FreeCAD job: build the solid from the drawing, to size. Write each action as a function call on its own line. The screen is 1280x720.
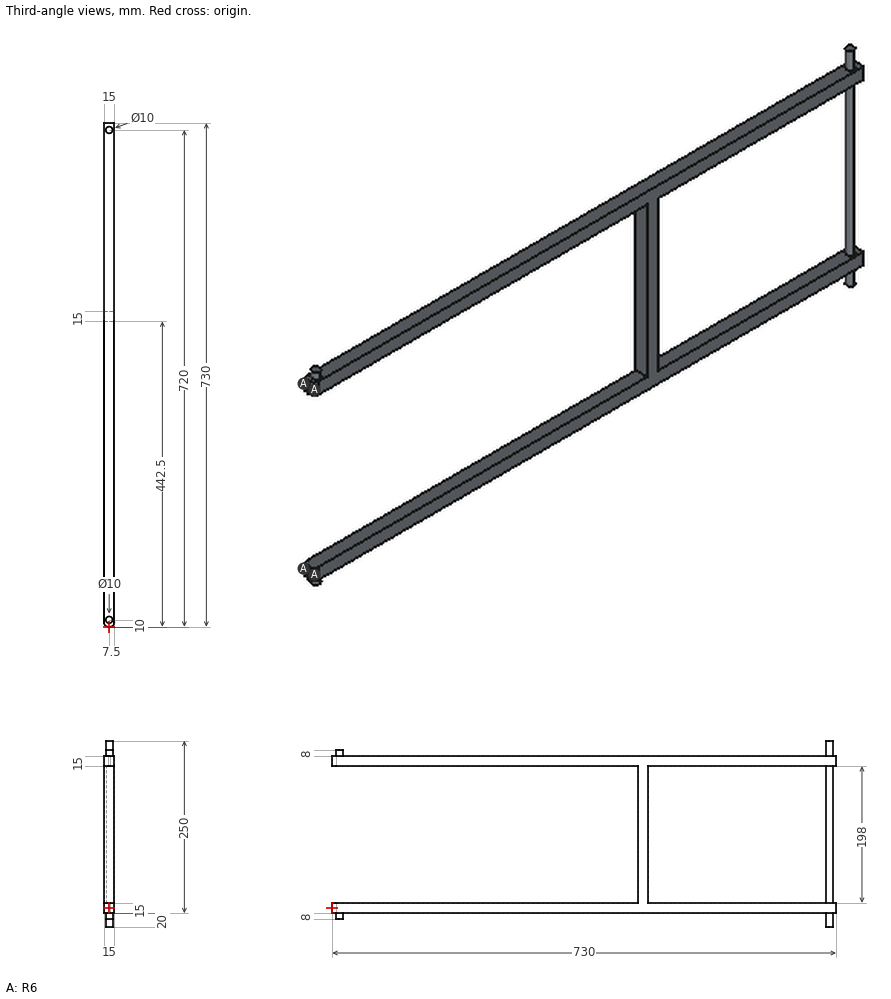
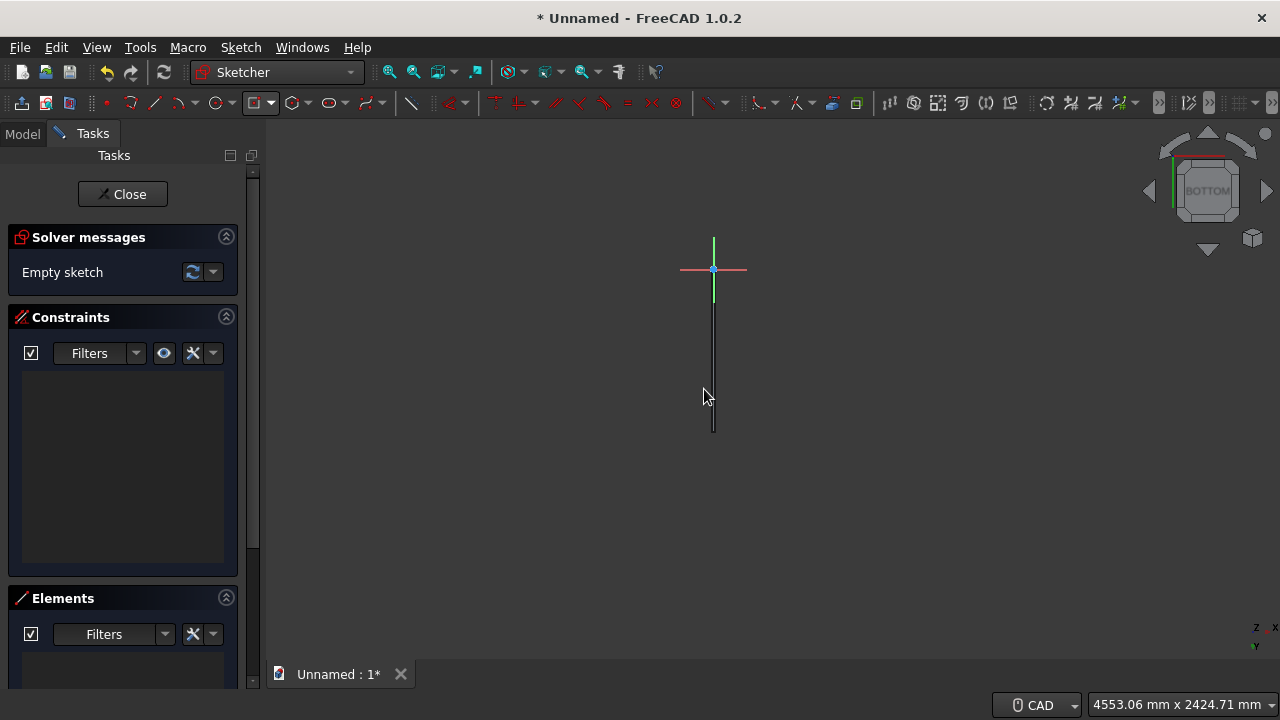
scroll(714, 265, up, 15)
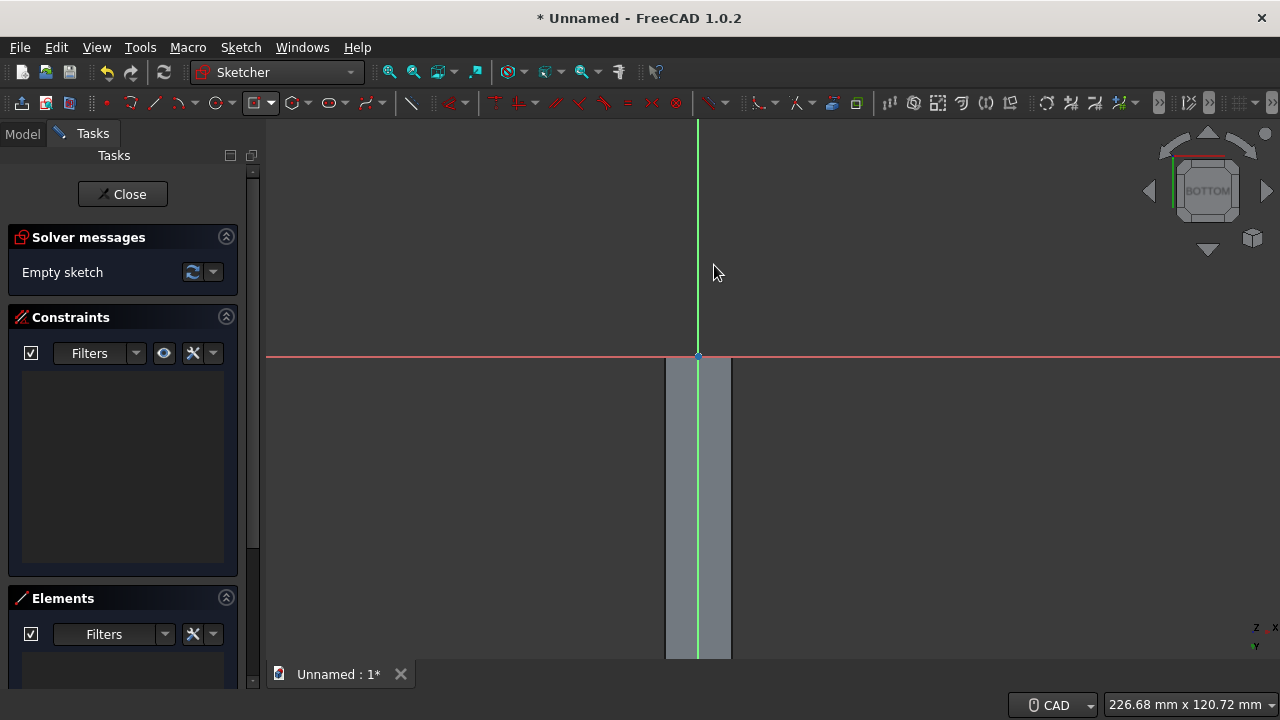
scroll(696, 390, up, 8)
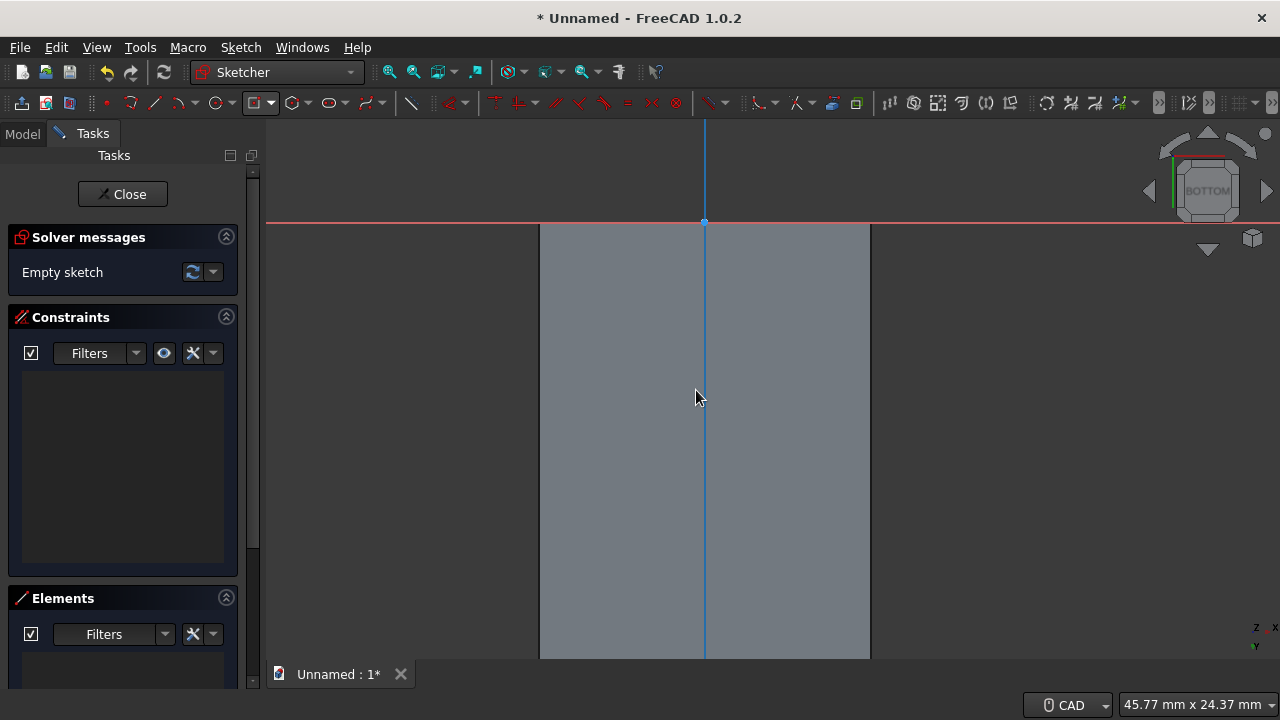
click(216, 104)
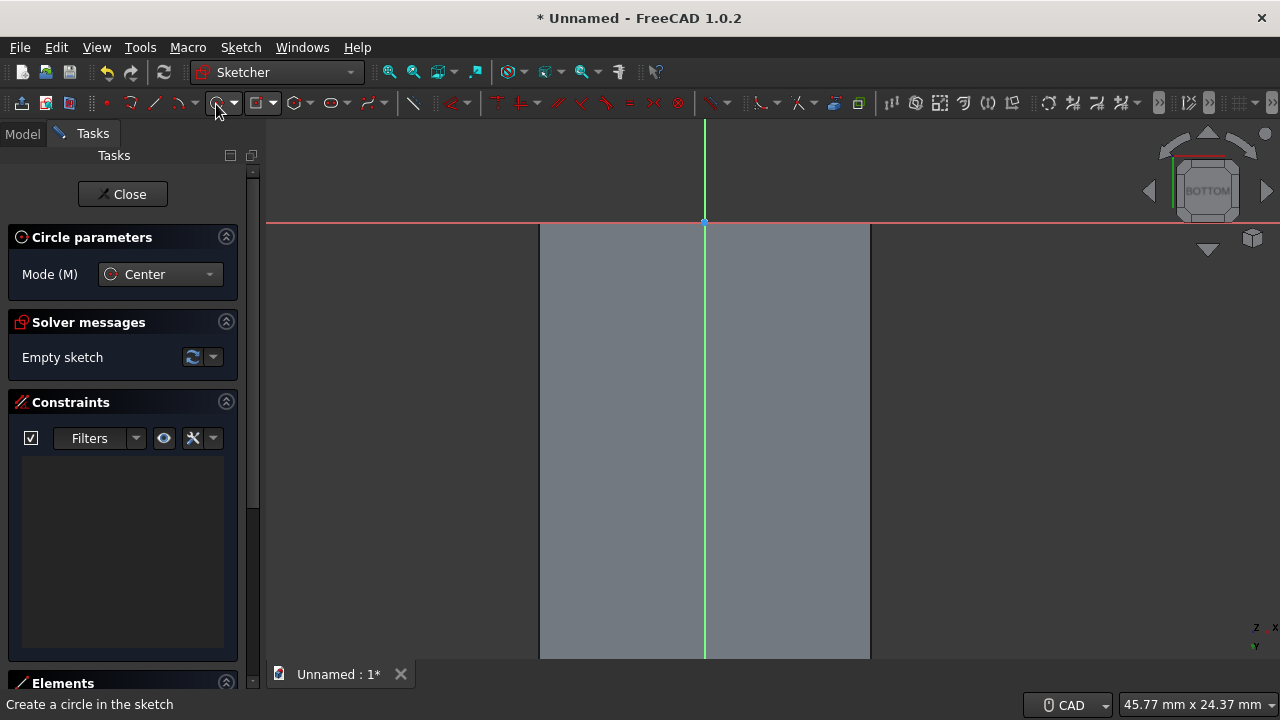
click(705, 444)
move(783, 366)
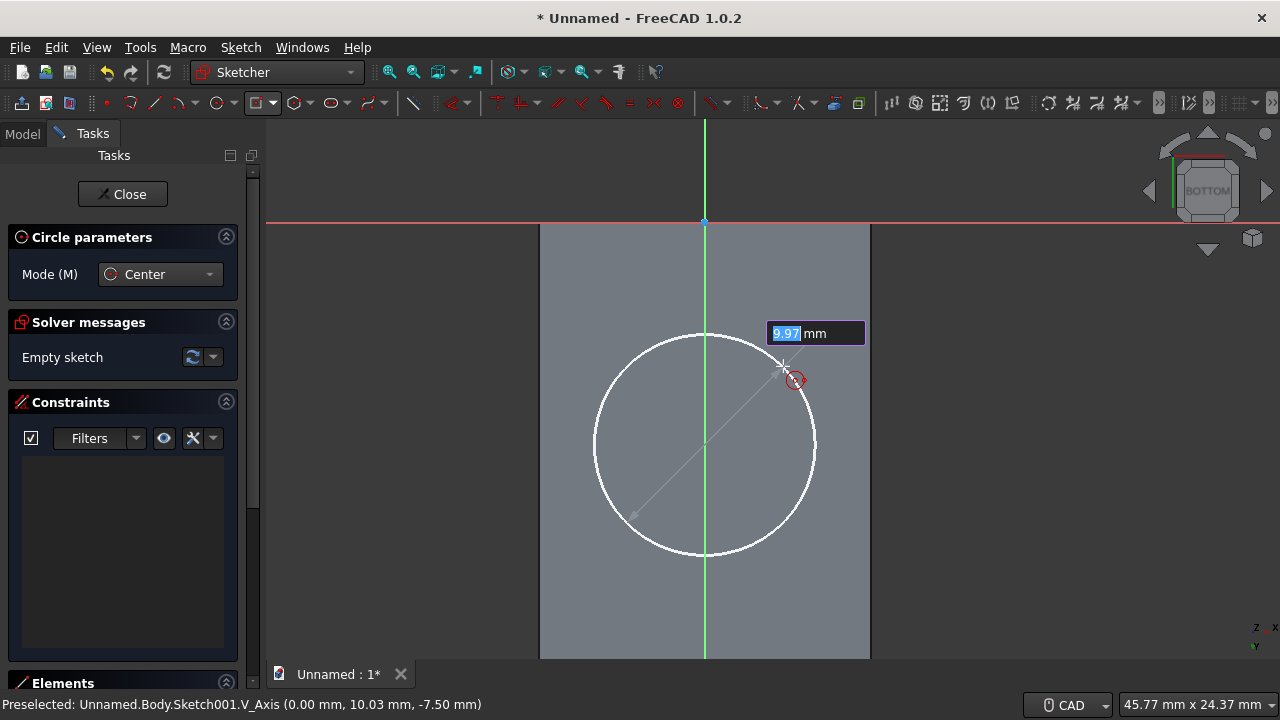
text(10)
key(Return)
key(Escape)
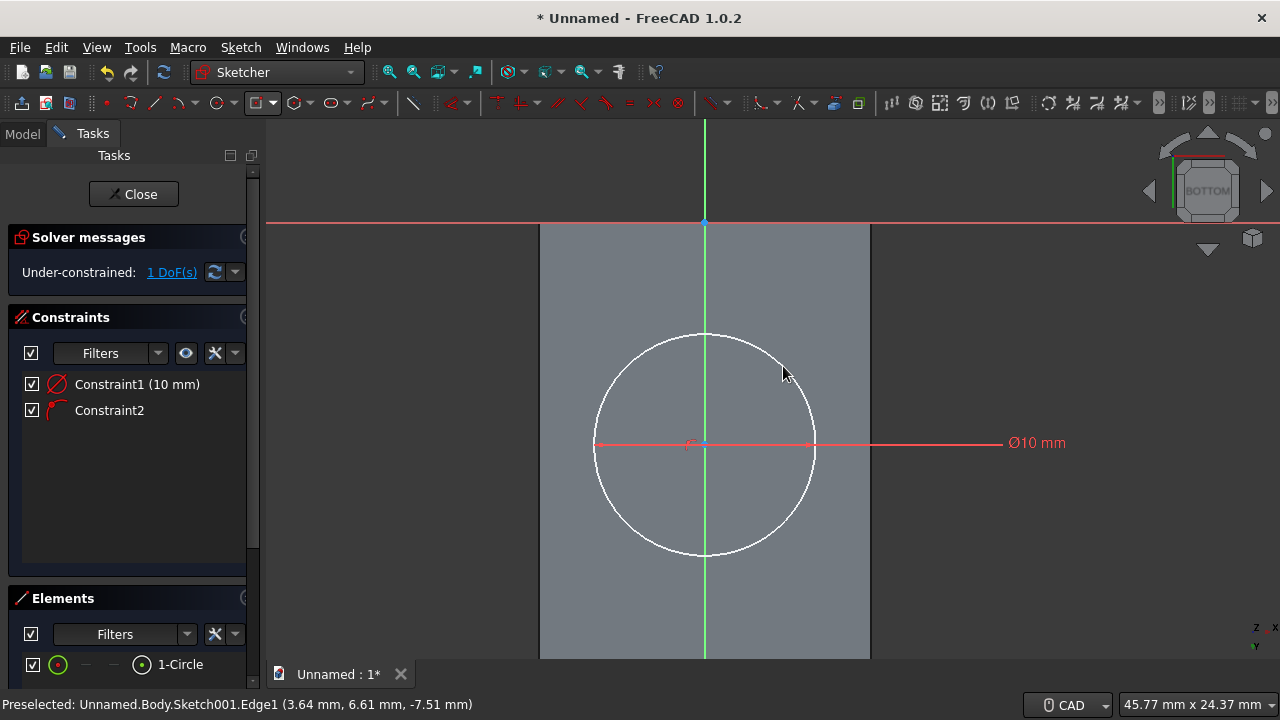
click(705, 445)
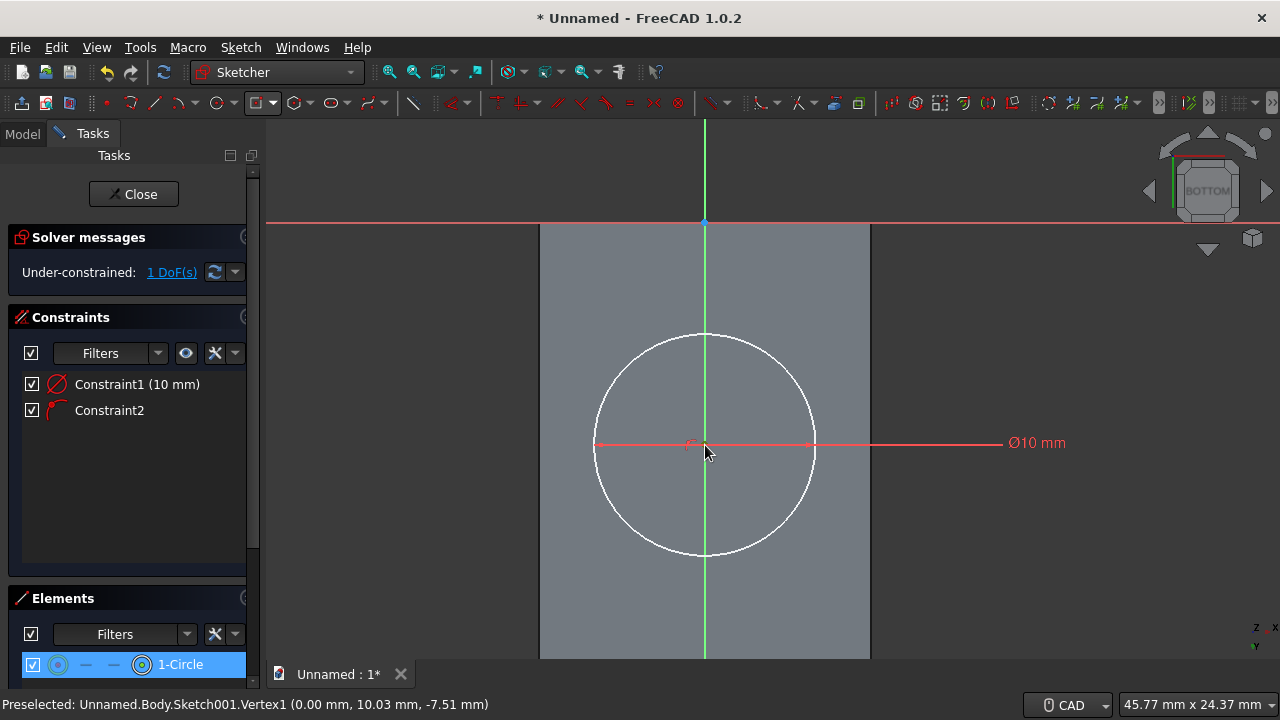
key(i)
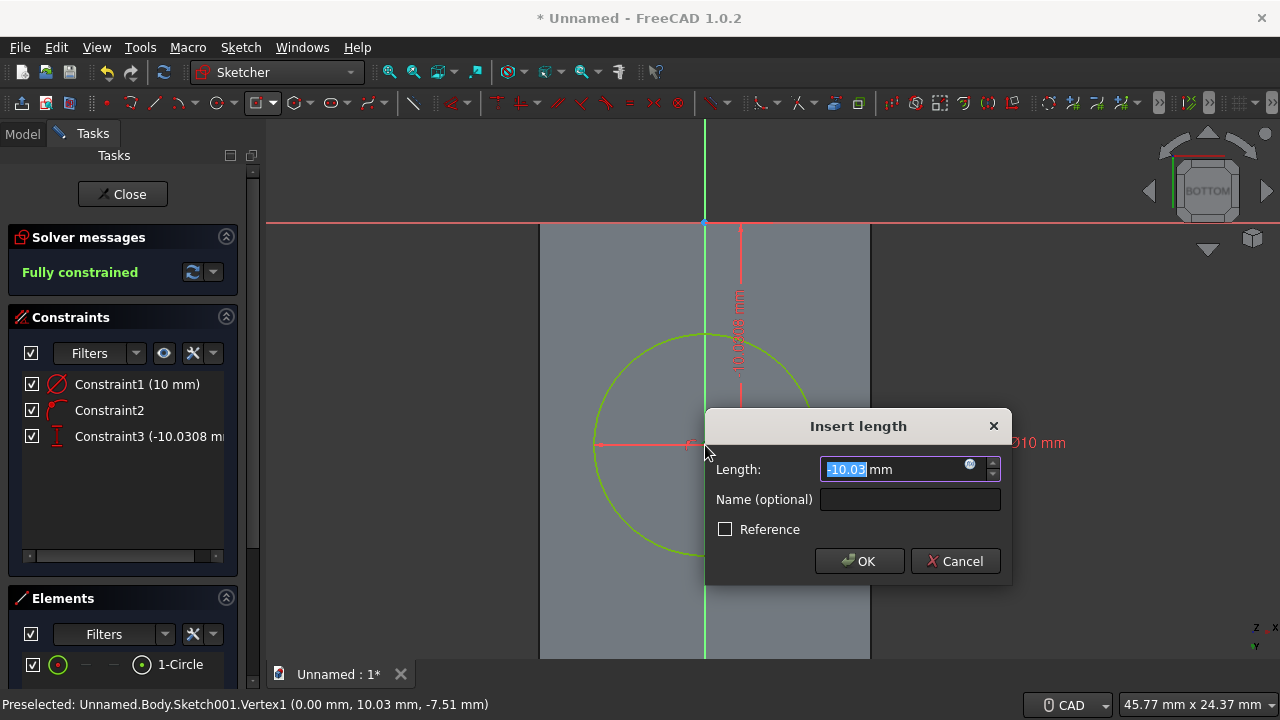
text(-10)
key(Return)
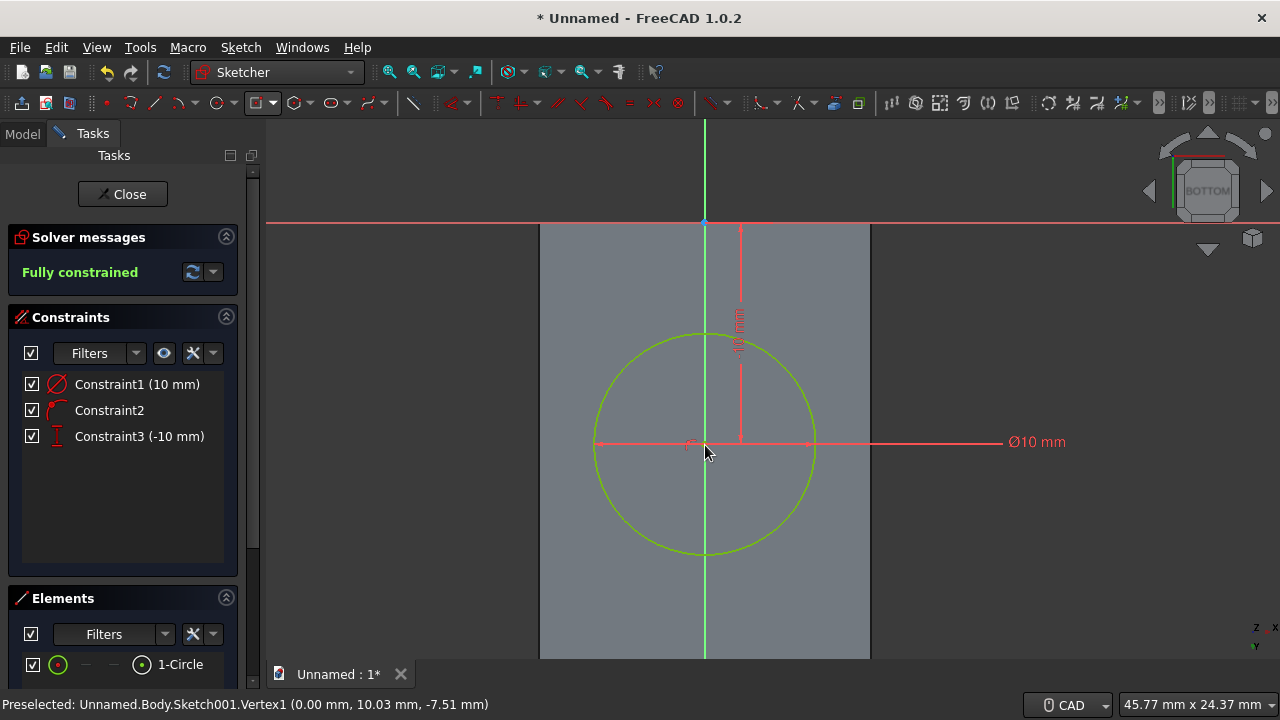
click(123, 194)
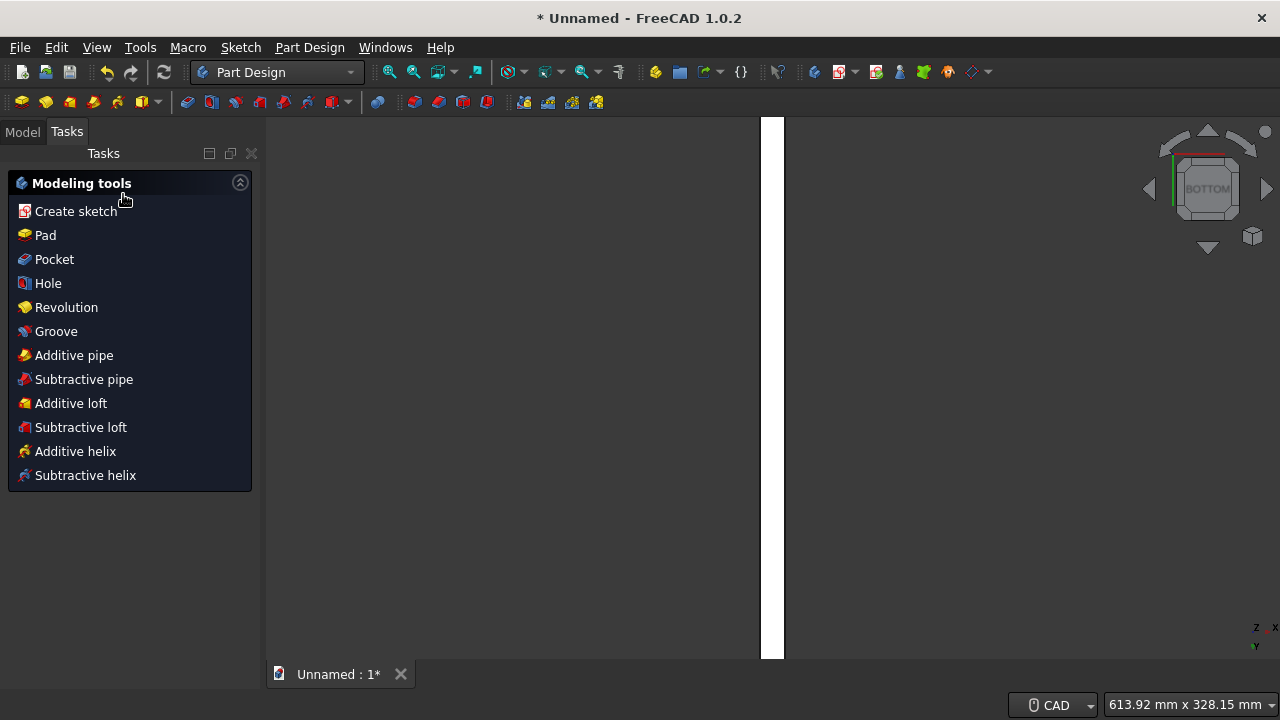
click(22, 102)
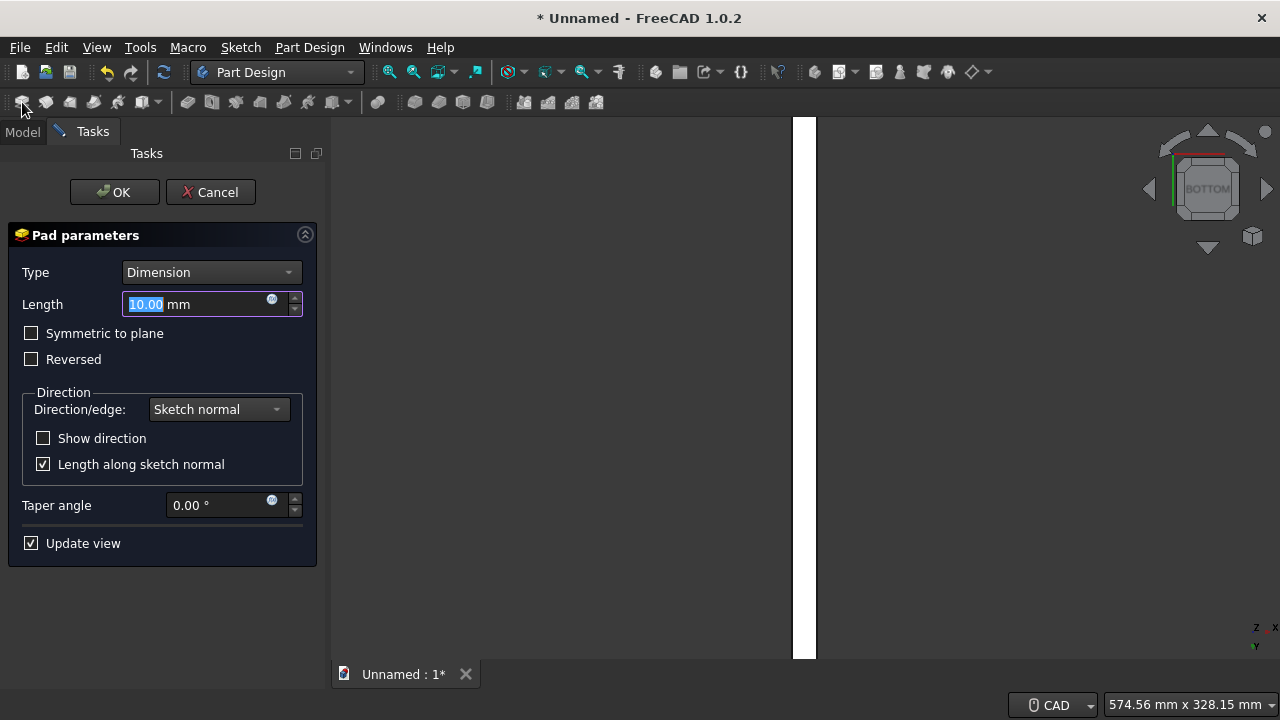
text(8)
key(Tab)